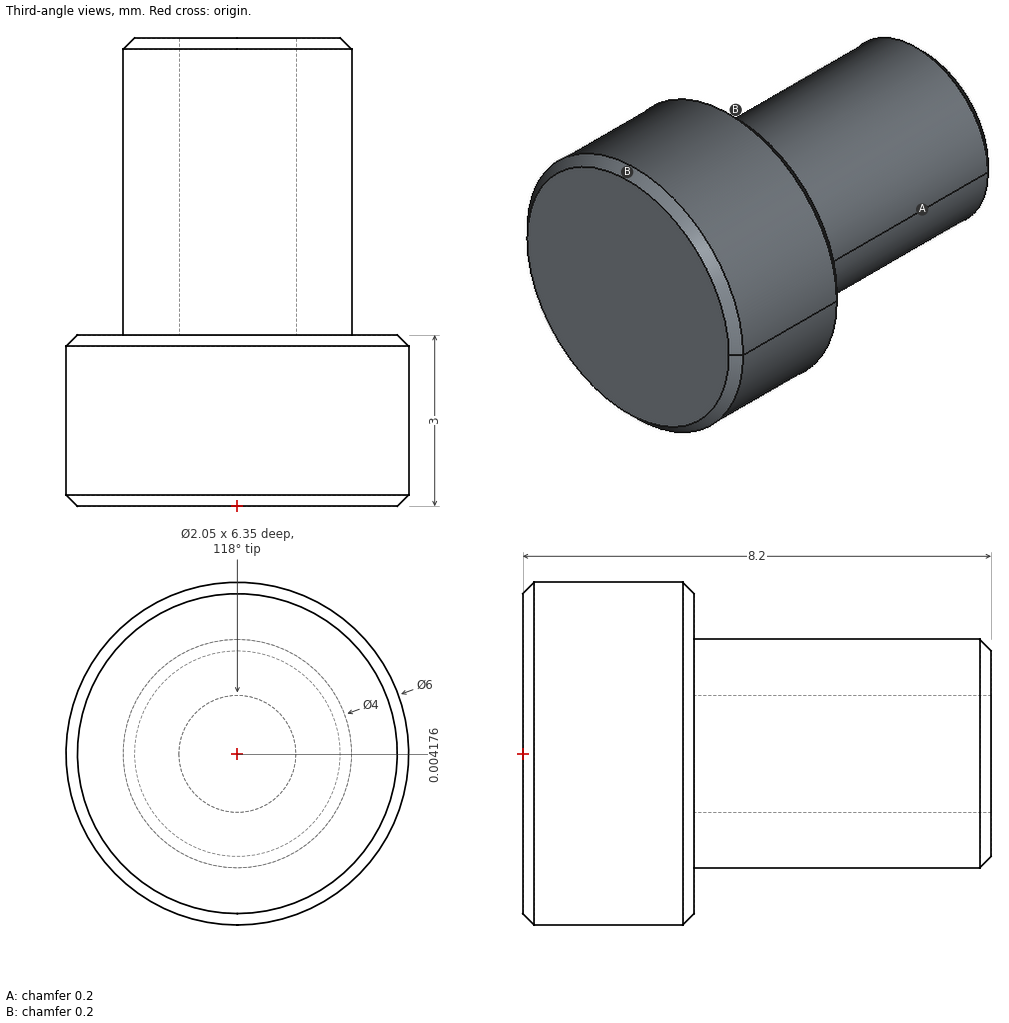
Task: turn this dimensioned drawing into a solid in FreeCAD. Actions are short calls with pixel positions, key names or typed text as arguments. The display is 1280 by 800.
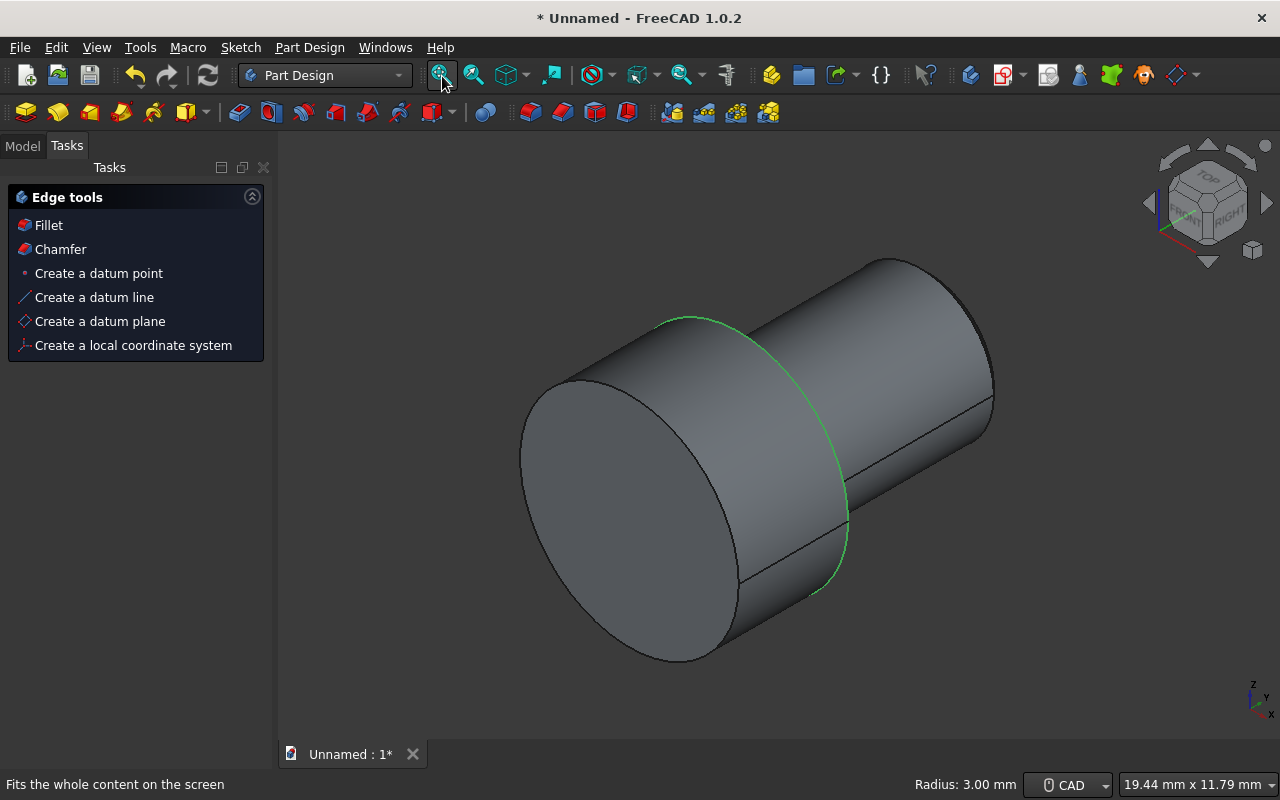
click(596, 381, ctrl)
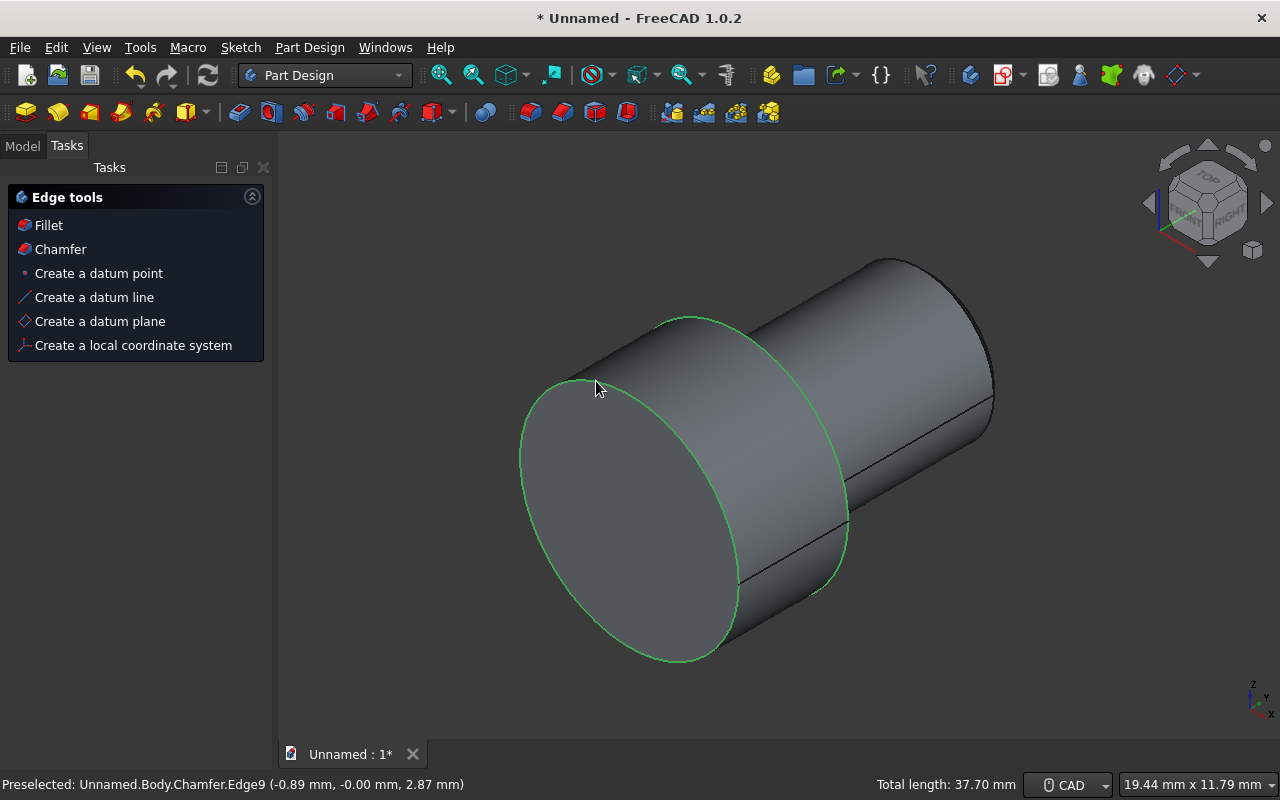
click(564, 112)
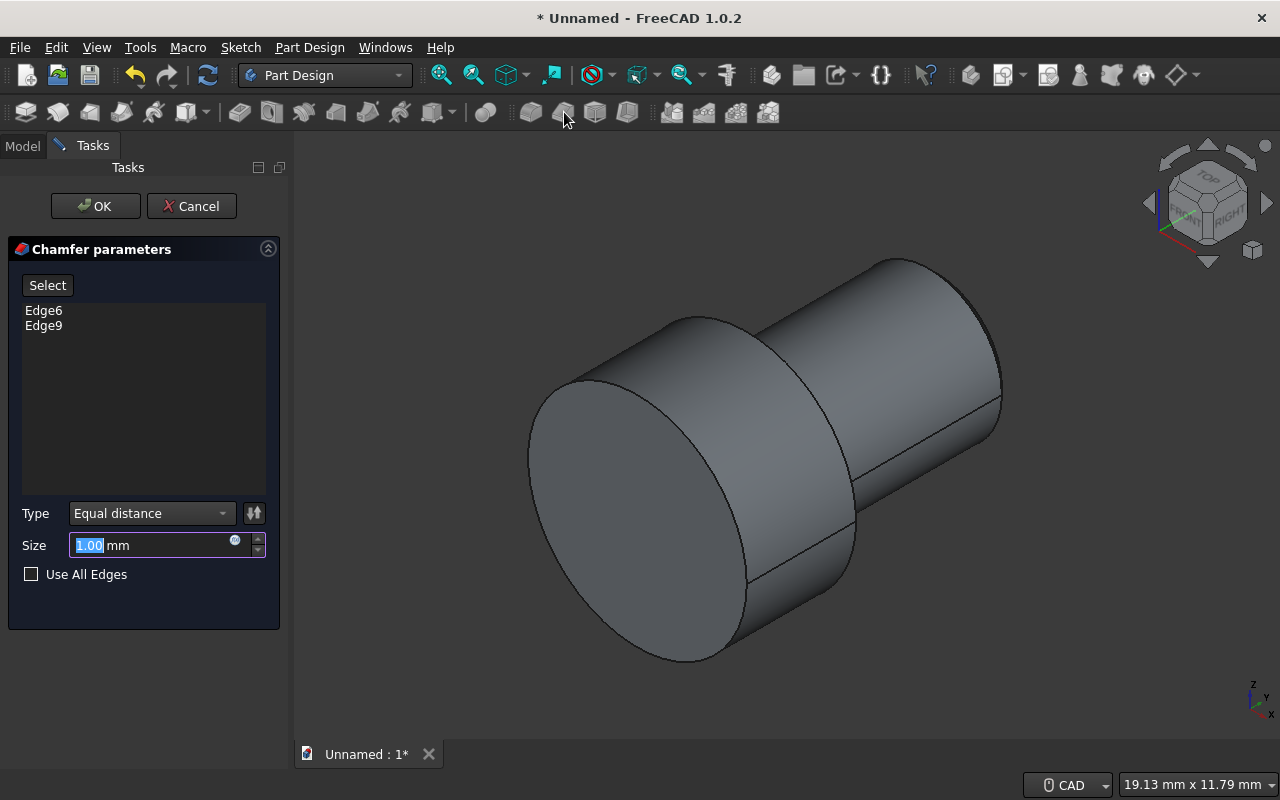
text(0.2)
key(Tab)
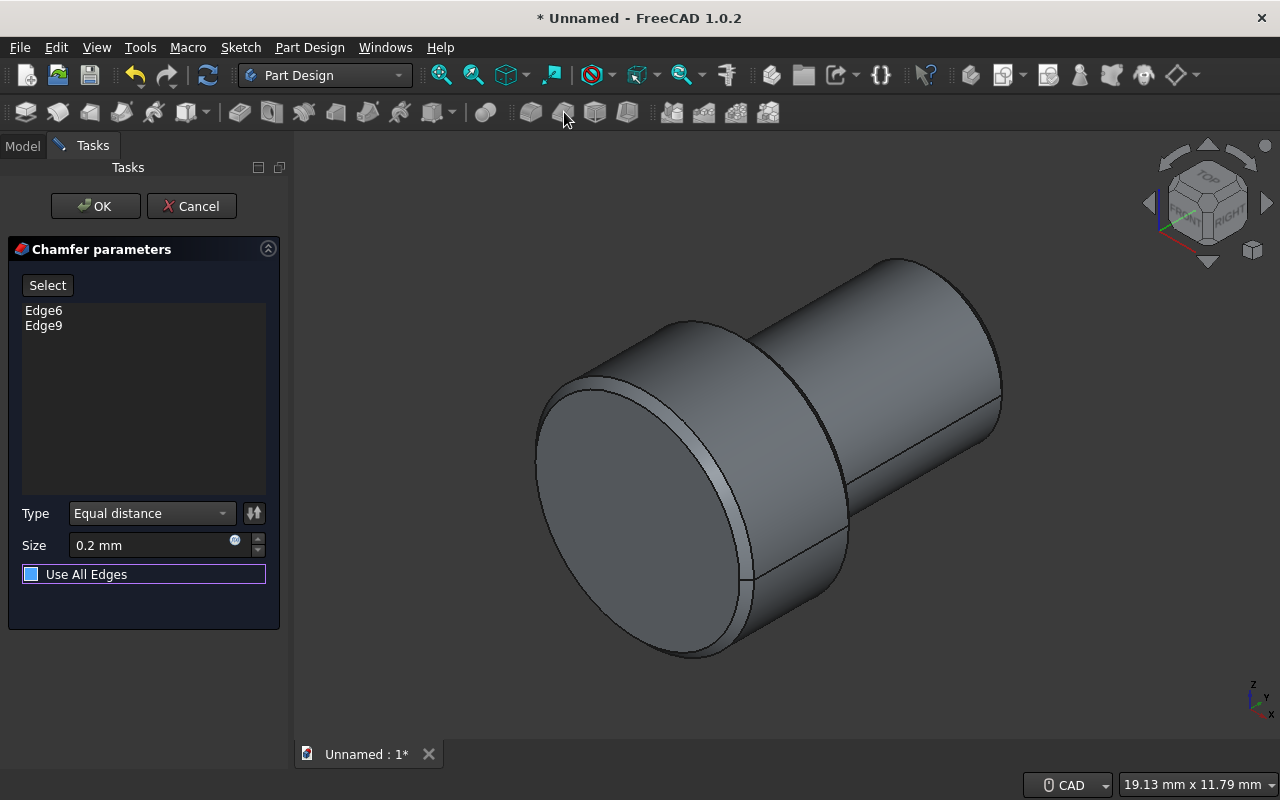
click(96, 206)